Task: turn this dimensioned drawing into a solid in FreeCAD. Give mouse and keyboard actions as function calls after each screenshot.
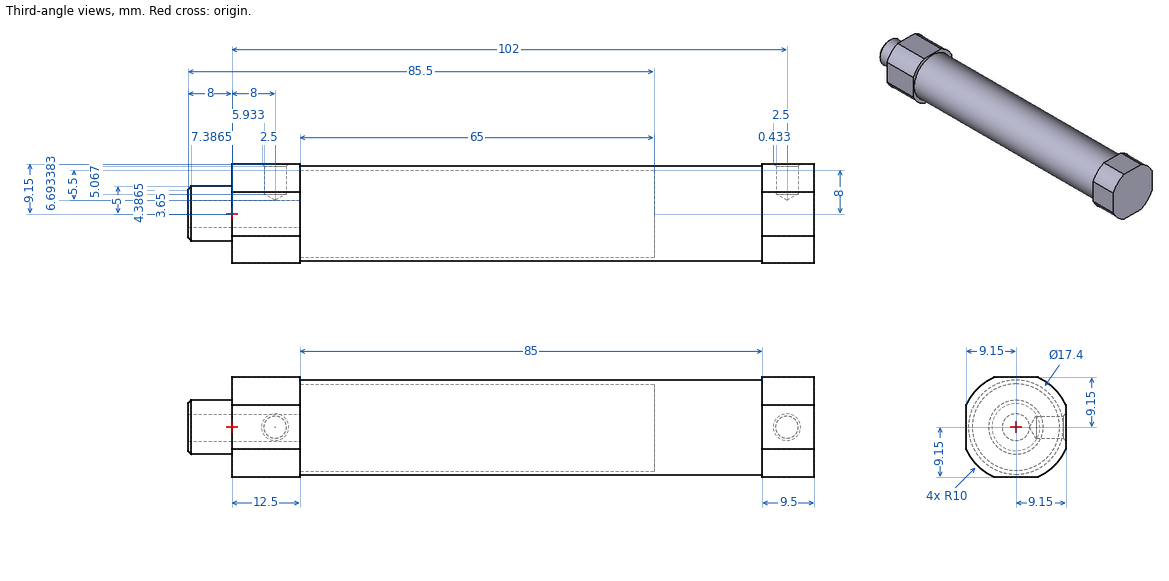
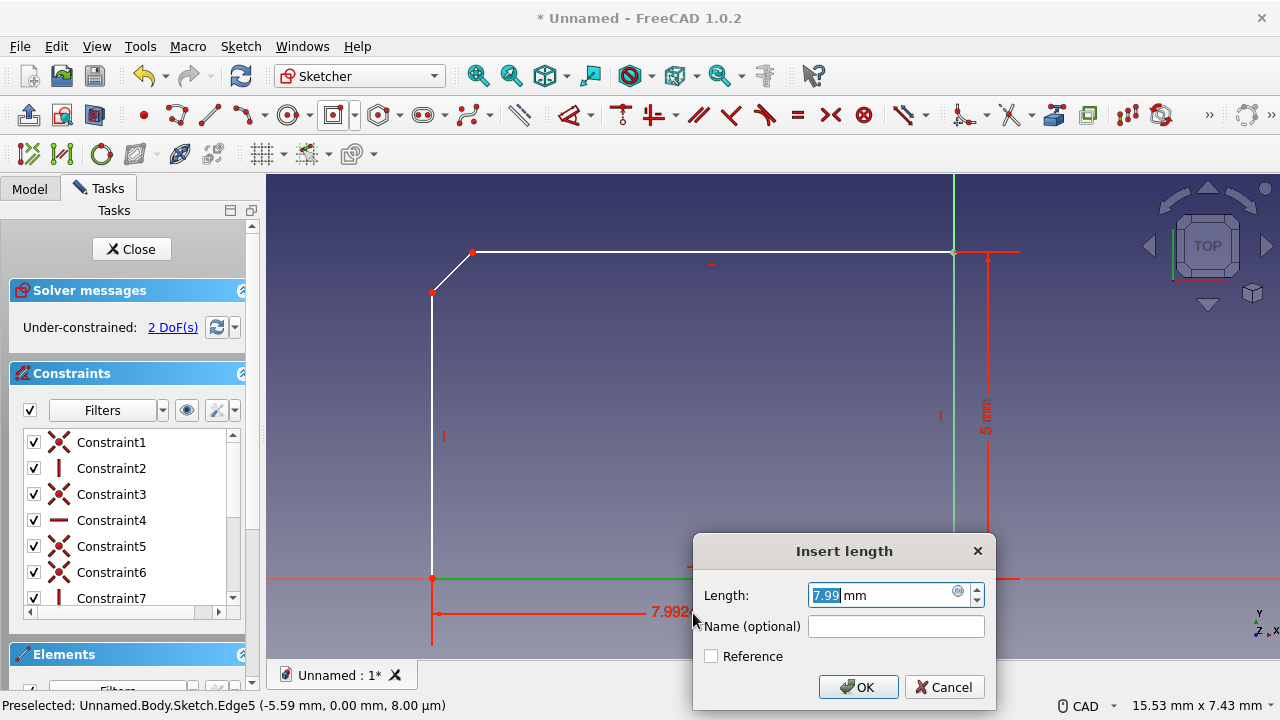
text(8)
key(Return)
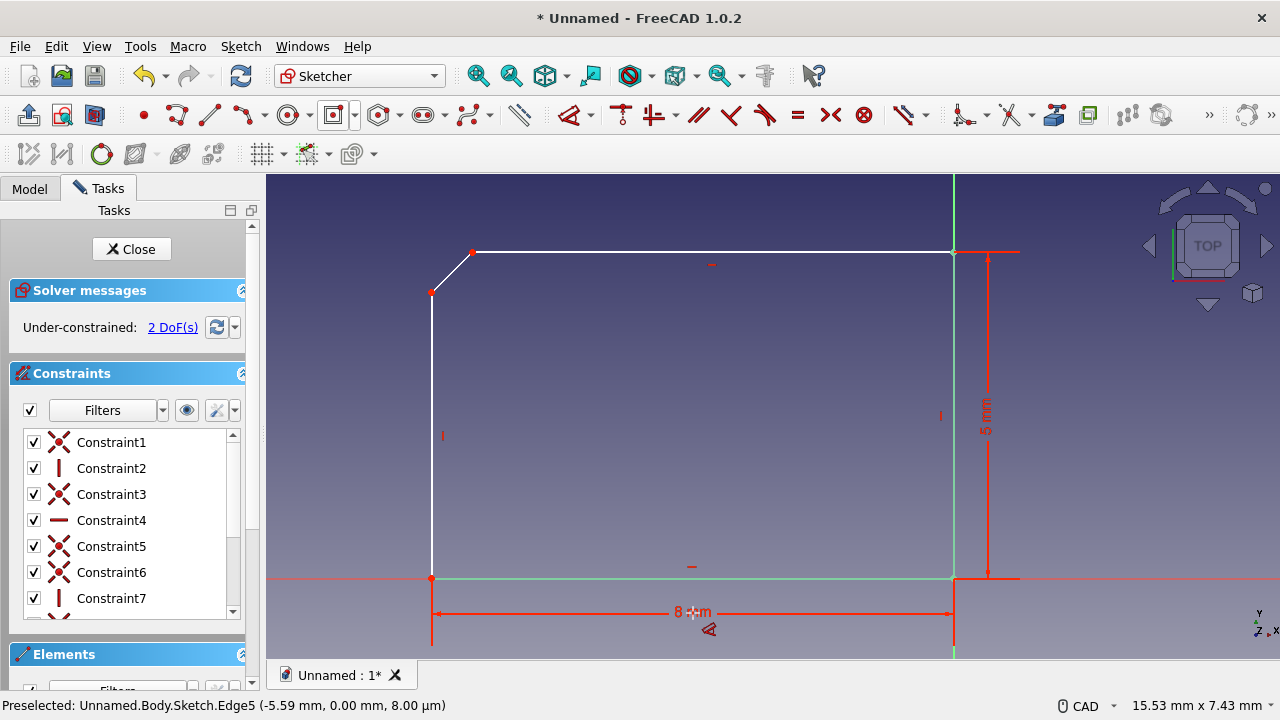
click(809, 252)
click(713, 218)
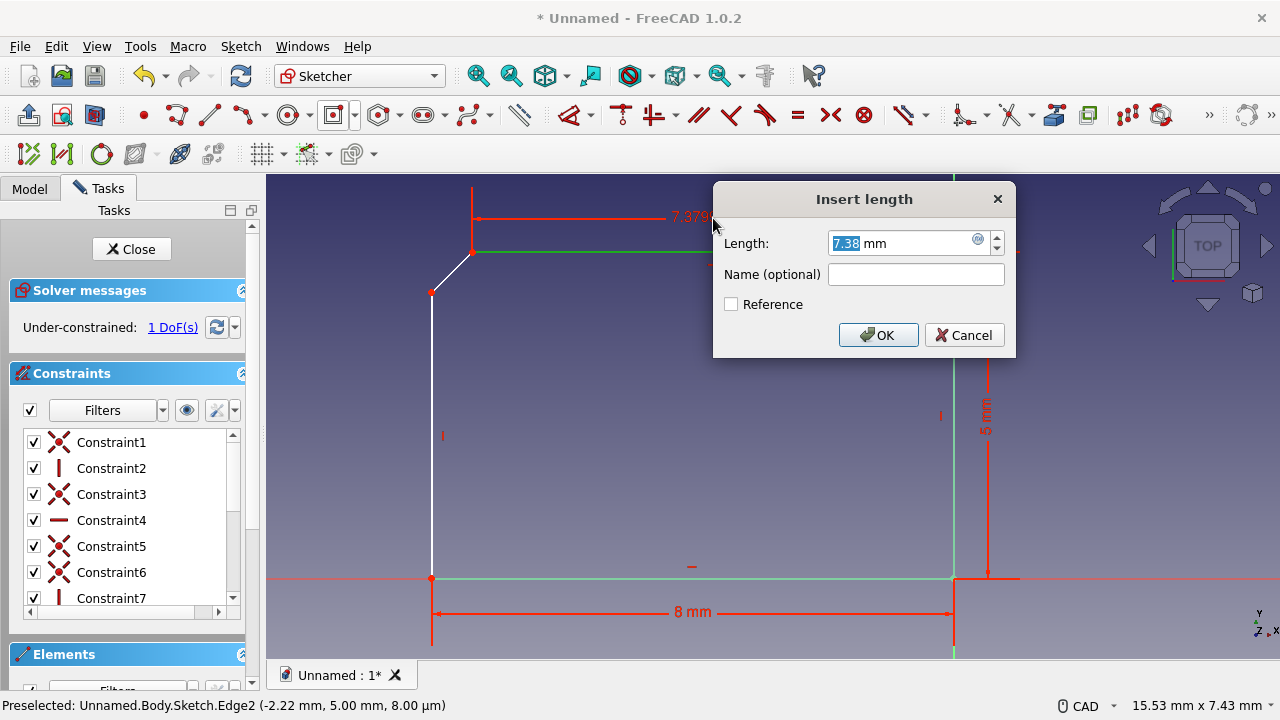
text(7.3865)
key(Return)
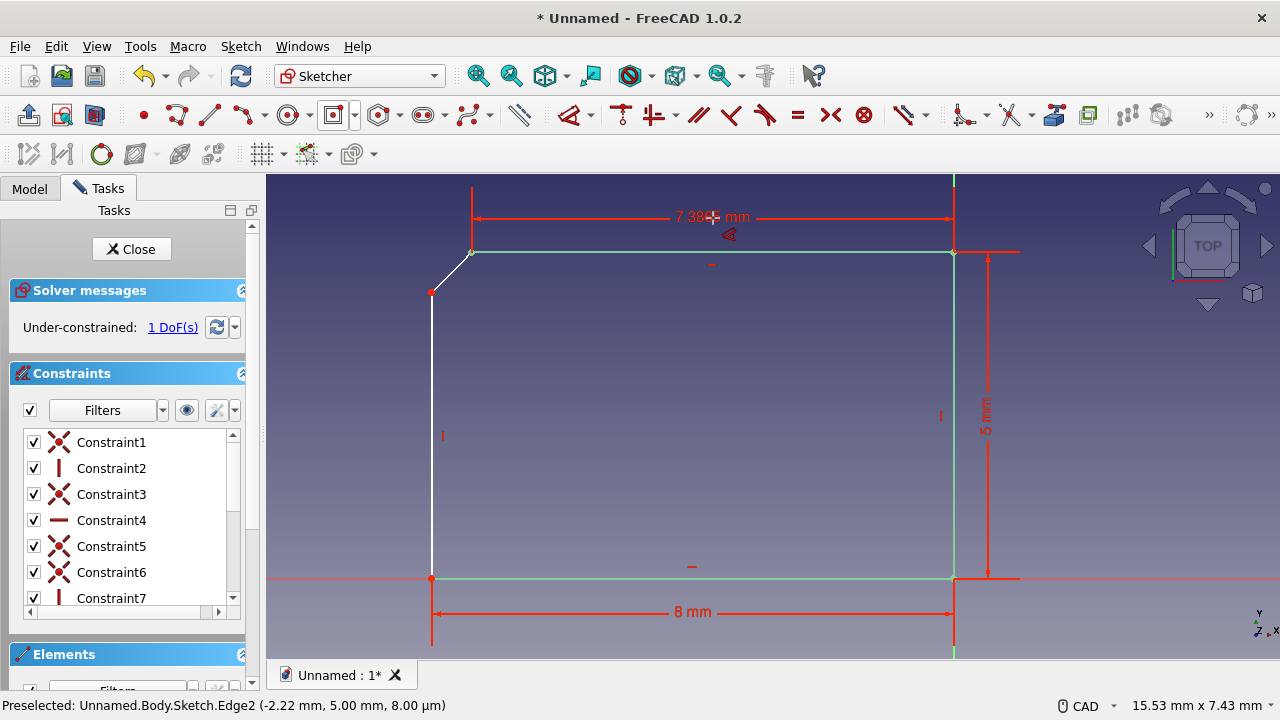
click(432, 379)
click(398, 436)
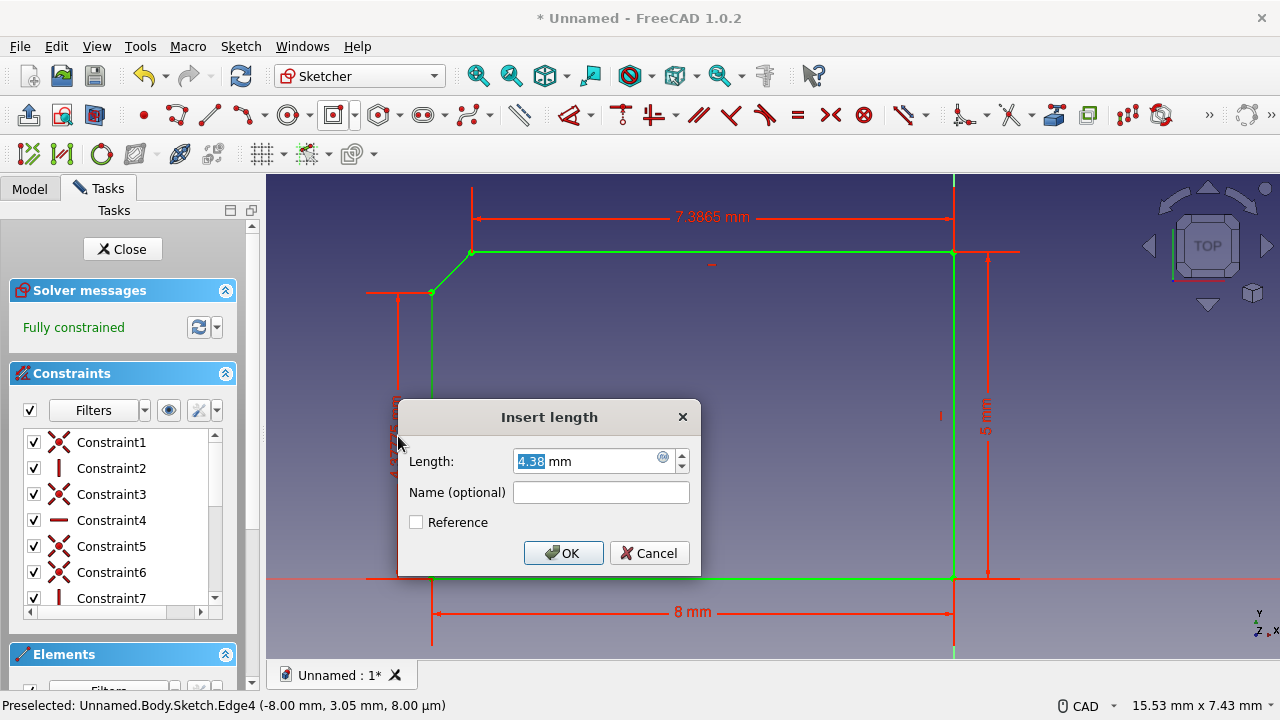
text(4.3865)
key(Return)
key(Escape)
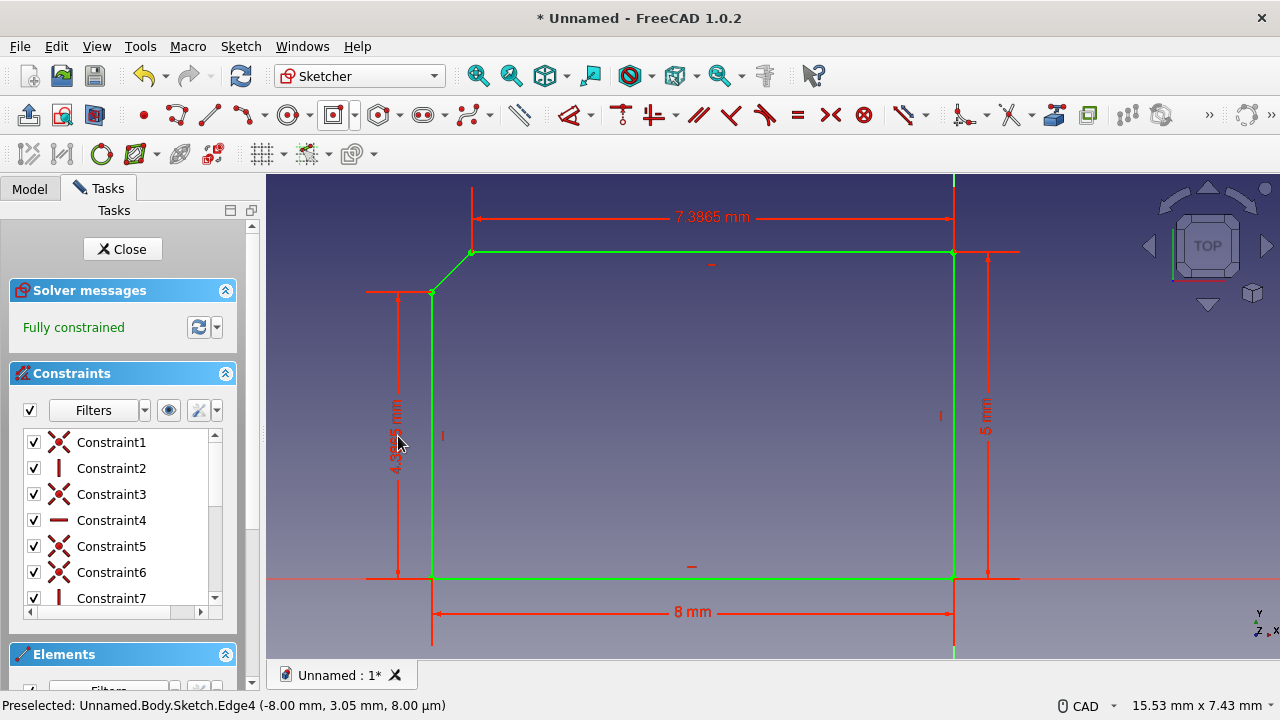
click(123, 249)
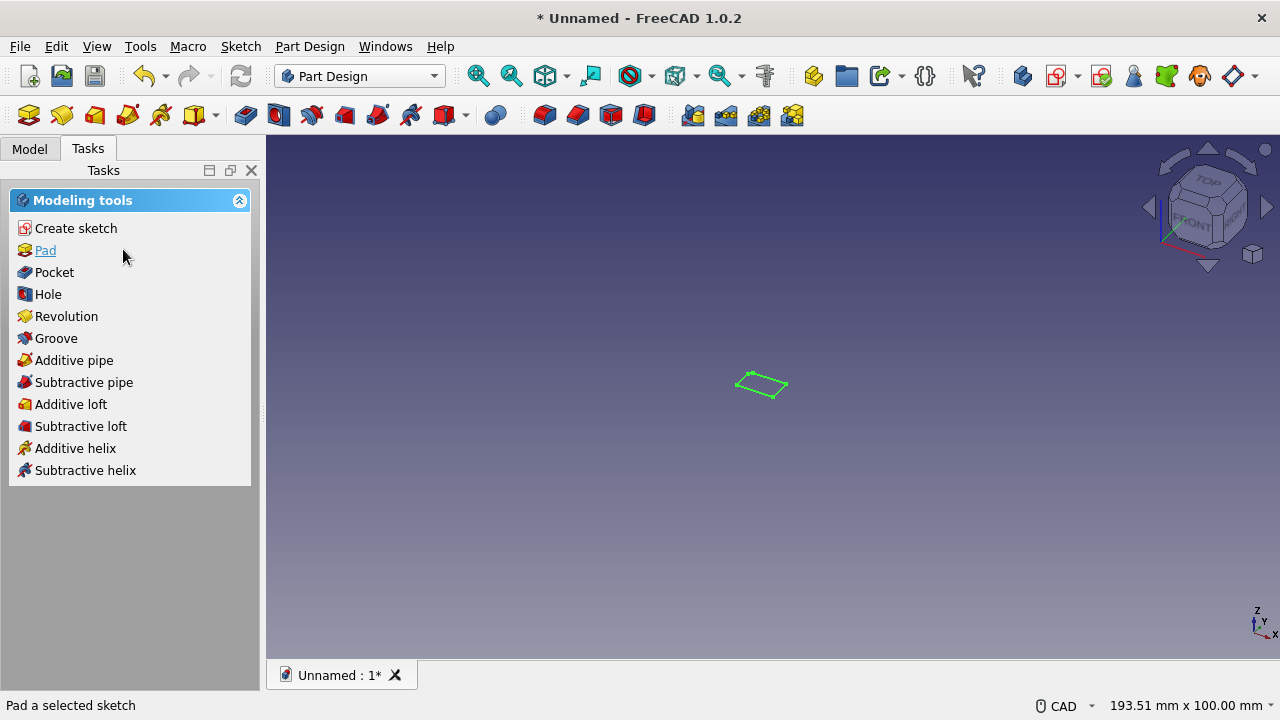
click(62, 116)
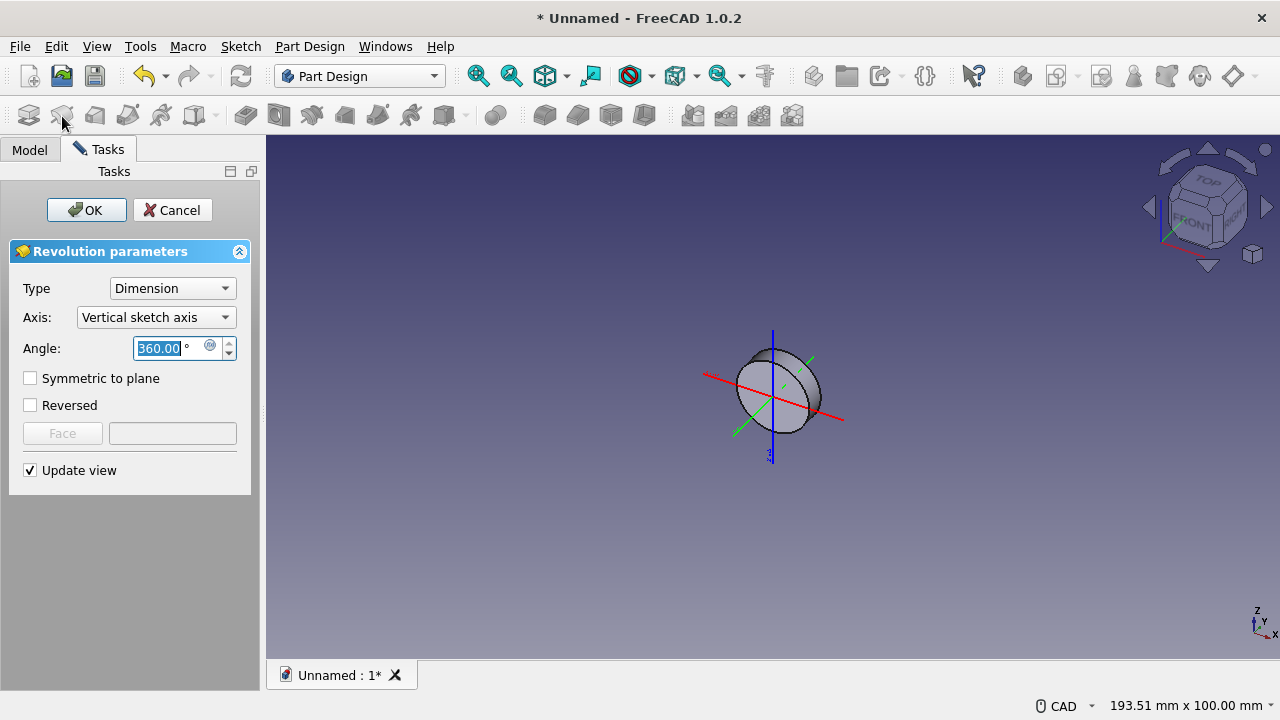
click(157, 318)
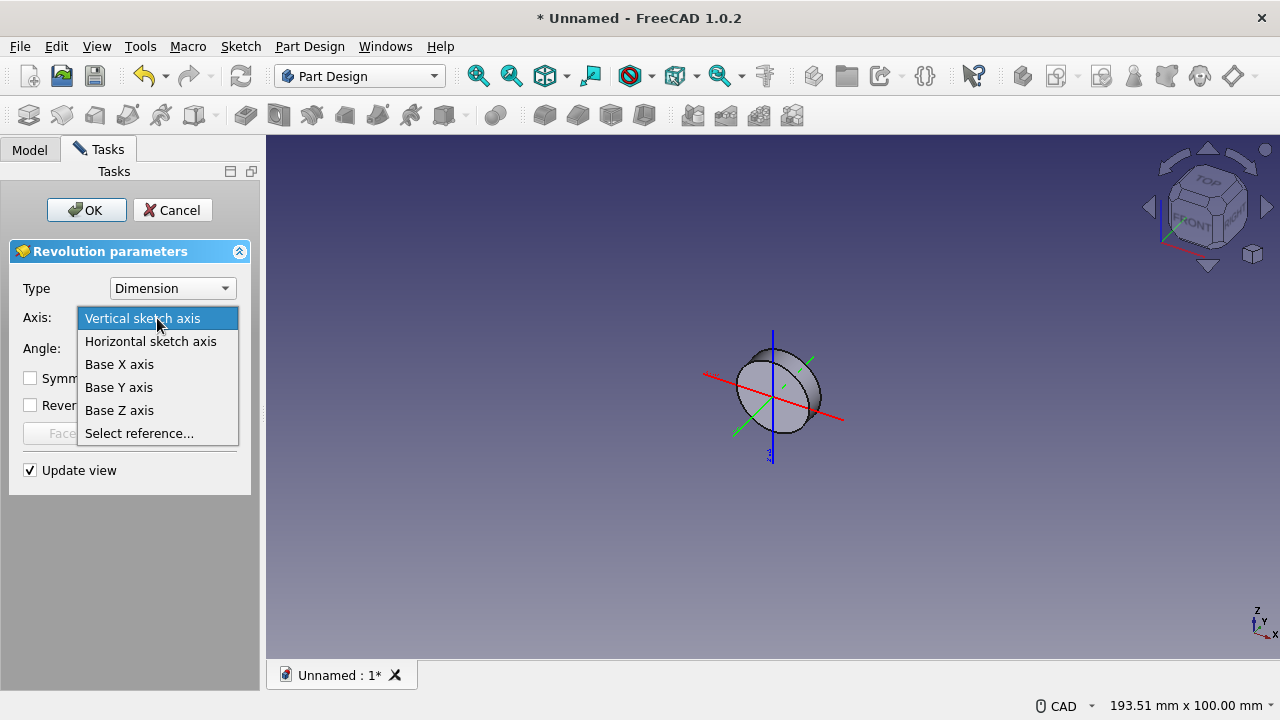
click(156, 342)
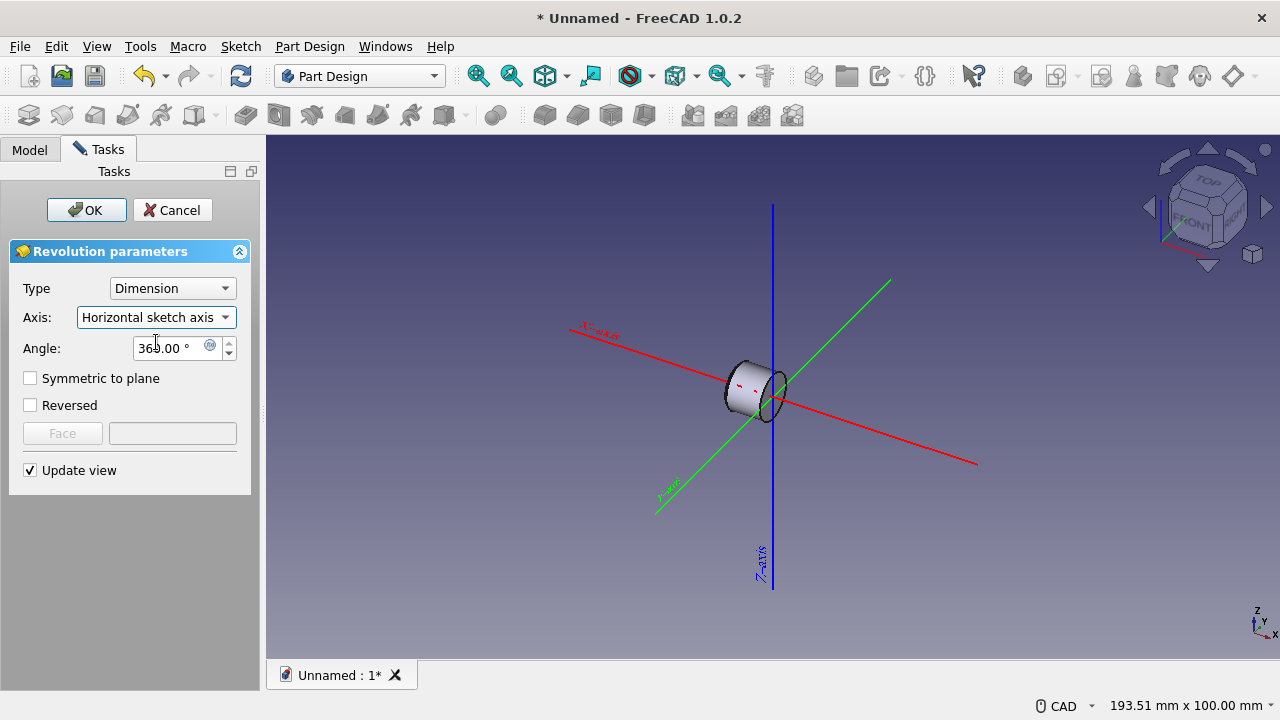
click(87, 210)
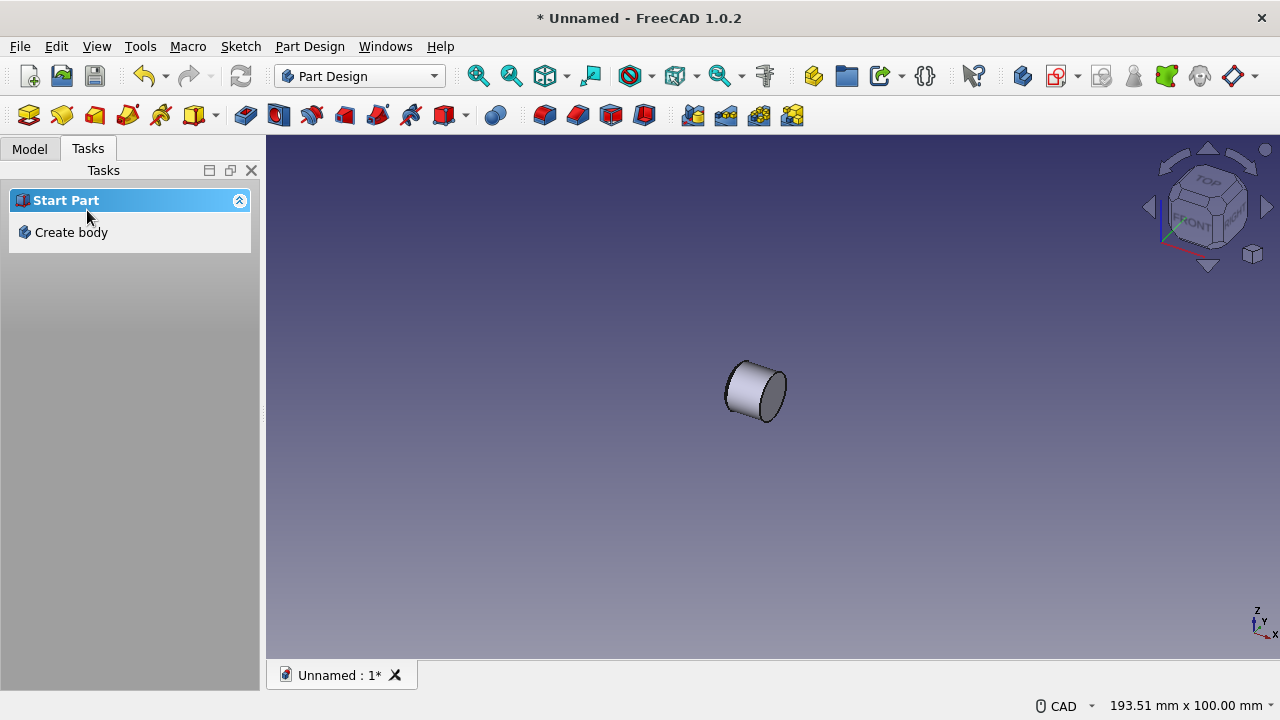
click(479, 76)